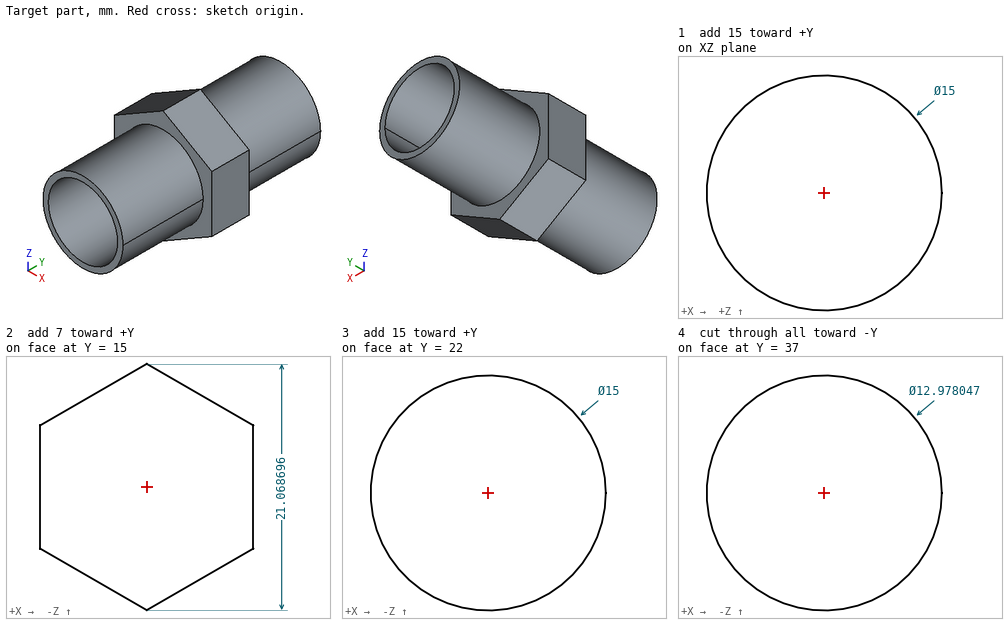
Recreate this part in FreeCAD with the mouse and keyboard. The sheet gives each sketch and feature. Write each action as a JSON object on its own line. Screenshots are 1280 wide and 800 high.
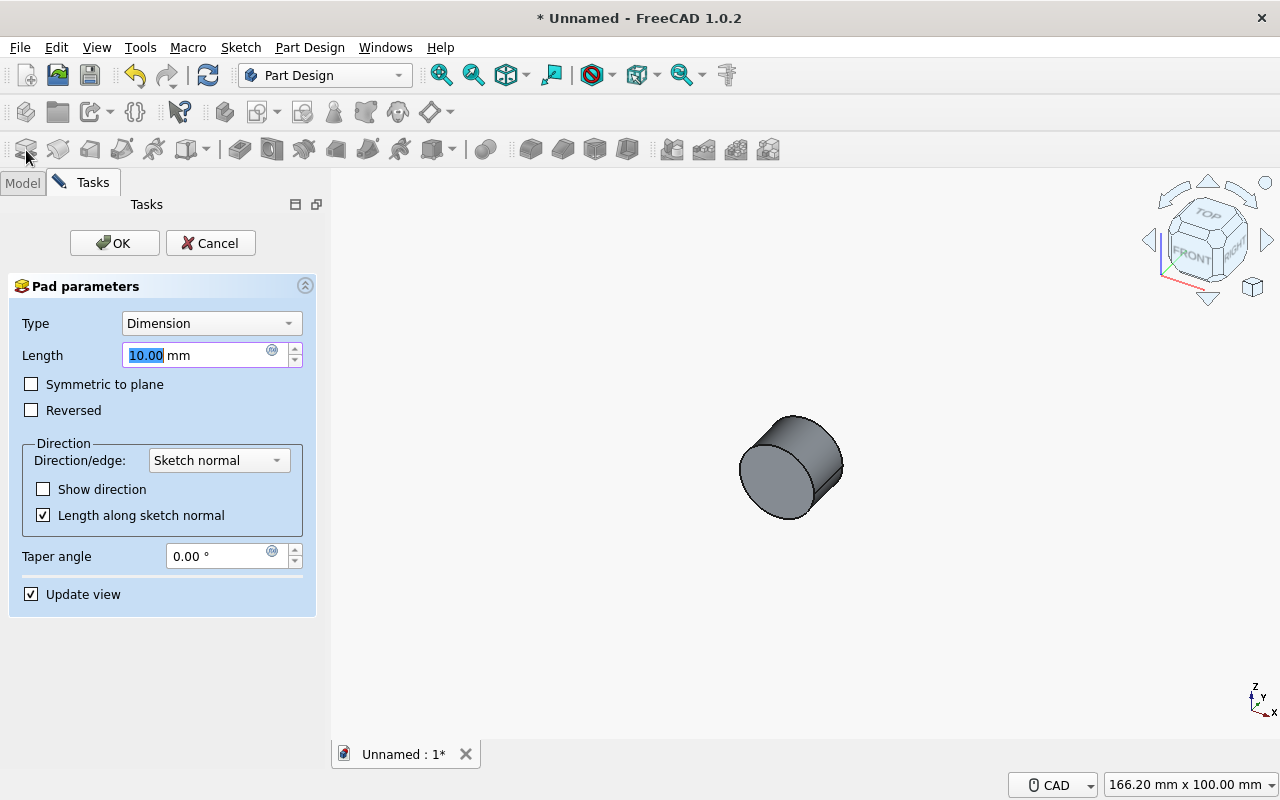
{"action": "type", "text": "15"}
{"action": "key", "text": "Tab"}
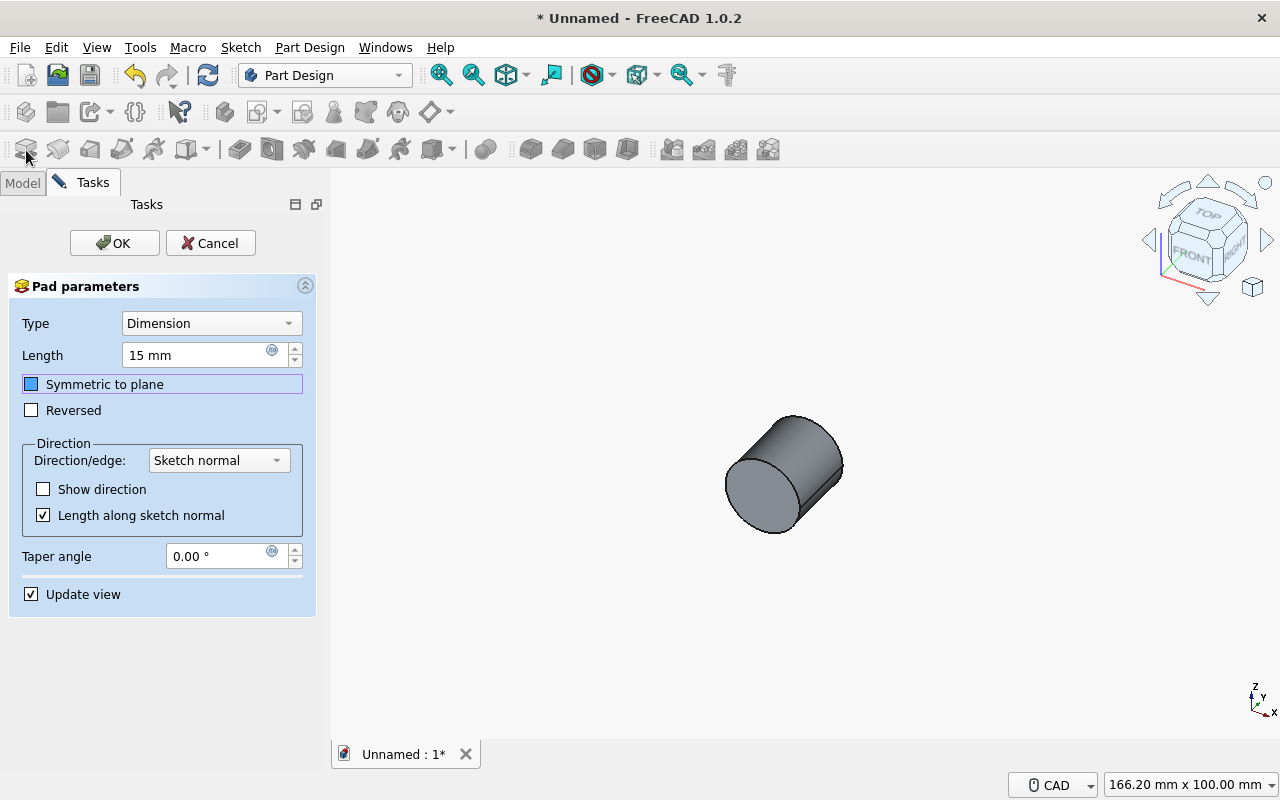
{"action": "left_click", "coordinate": [30, 410]}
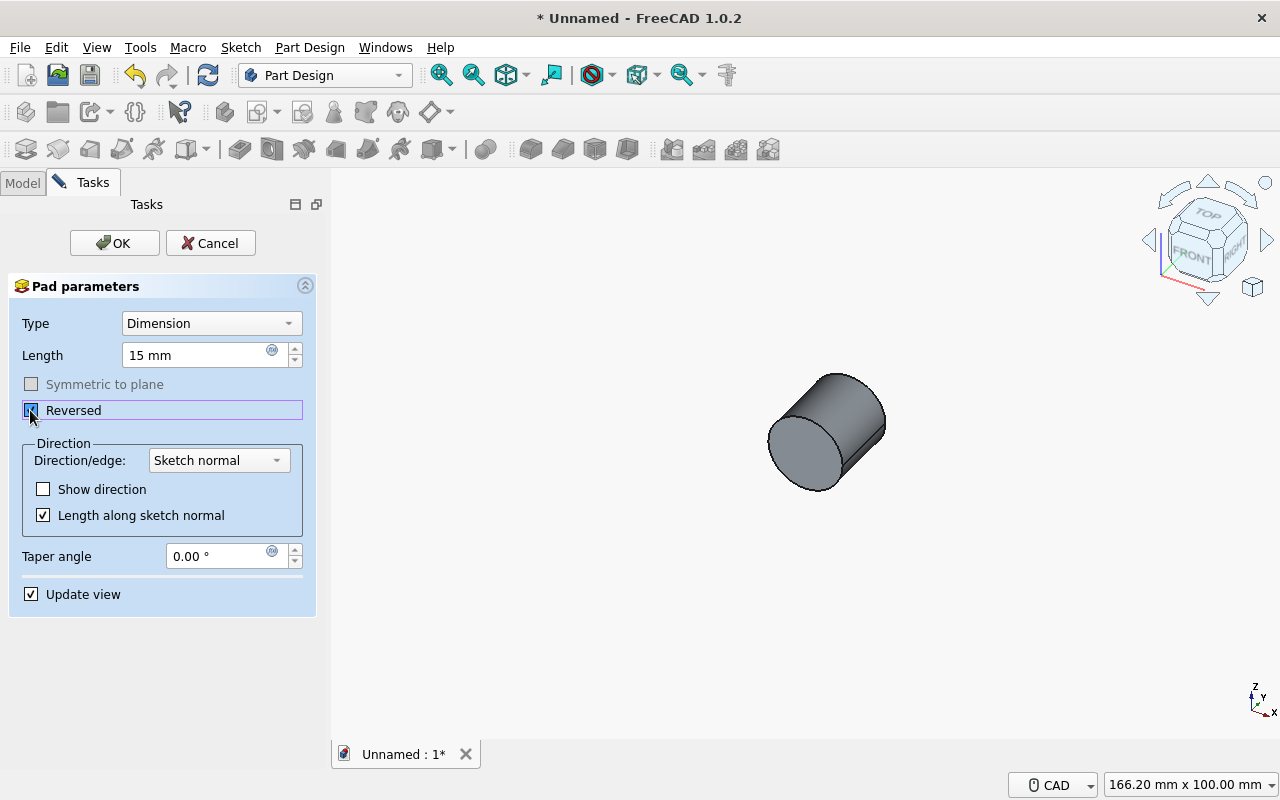
{"action": "left_click", "coordinate": [115, 243]}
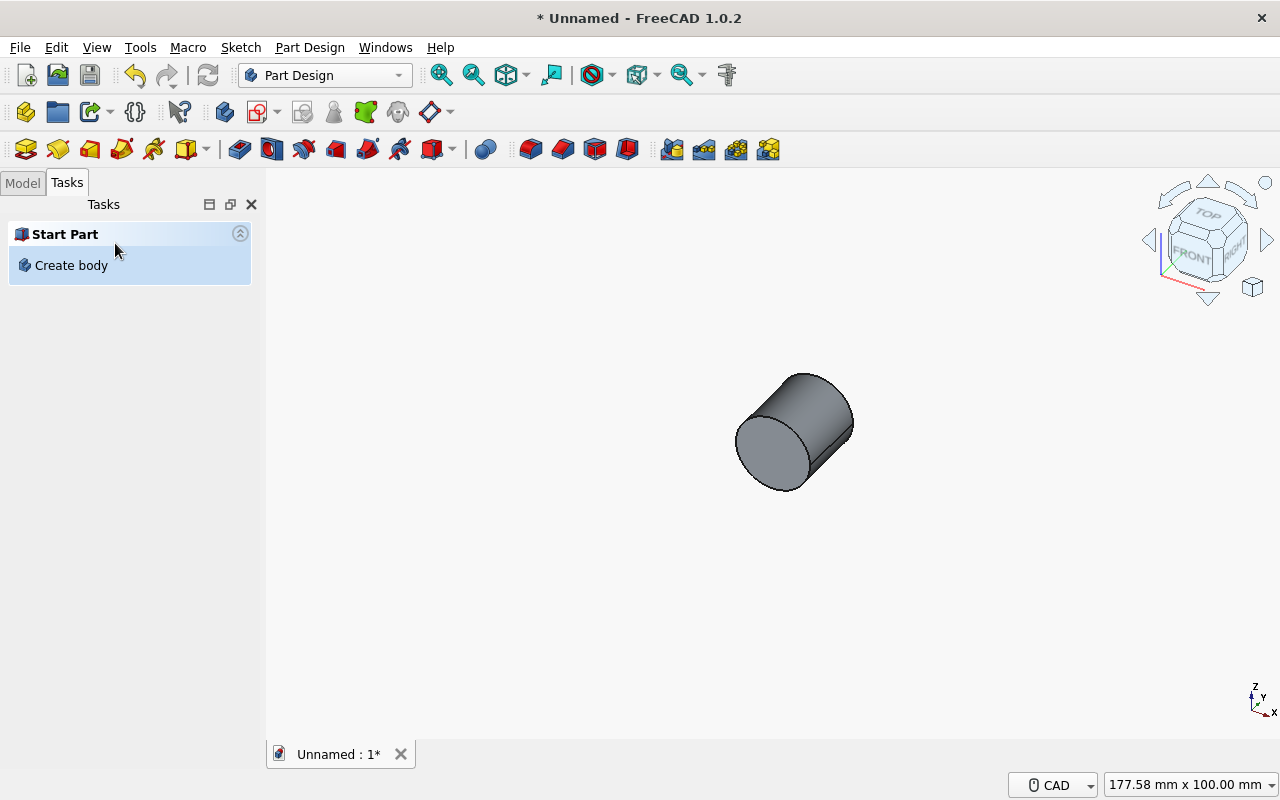
{"action": "left_click", "coordinate": [442, 76]}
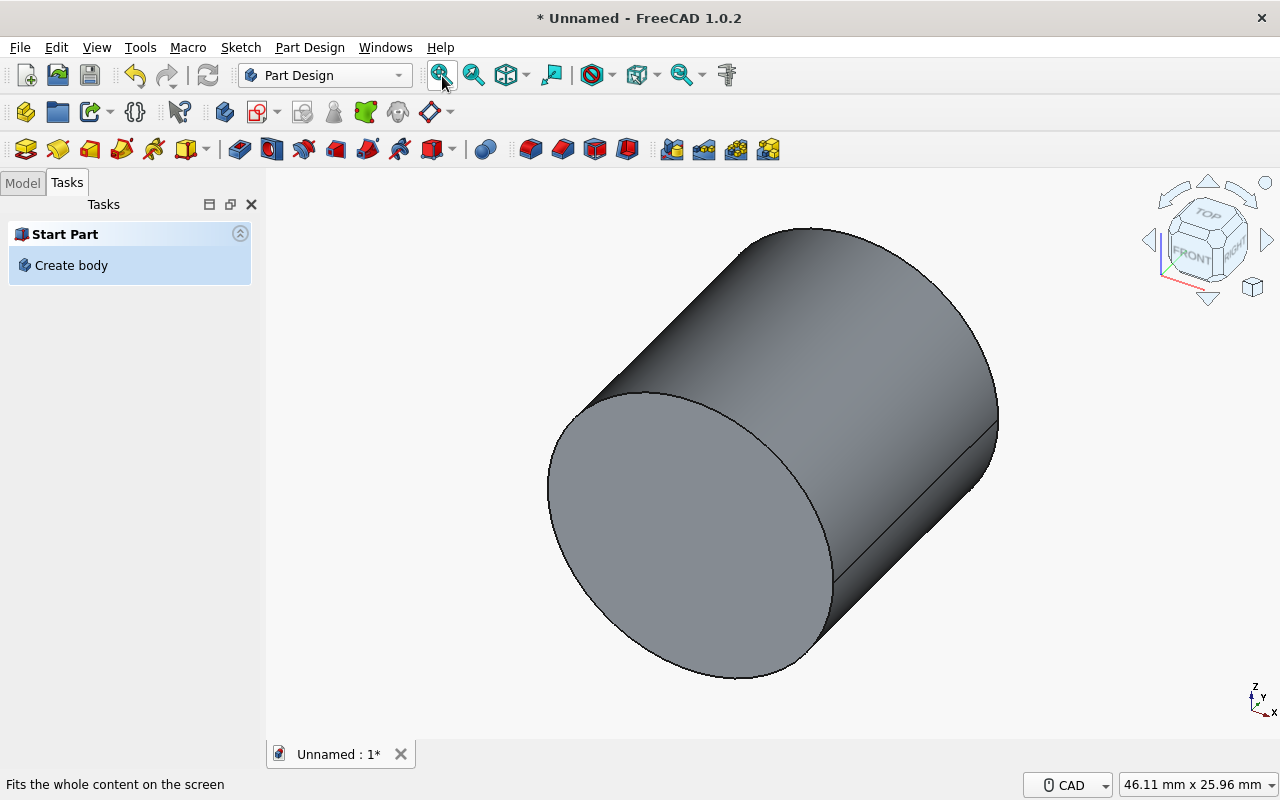
{"action": "key", "text": "4"}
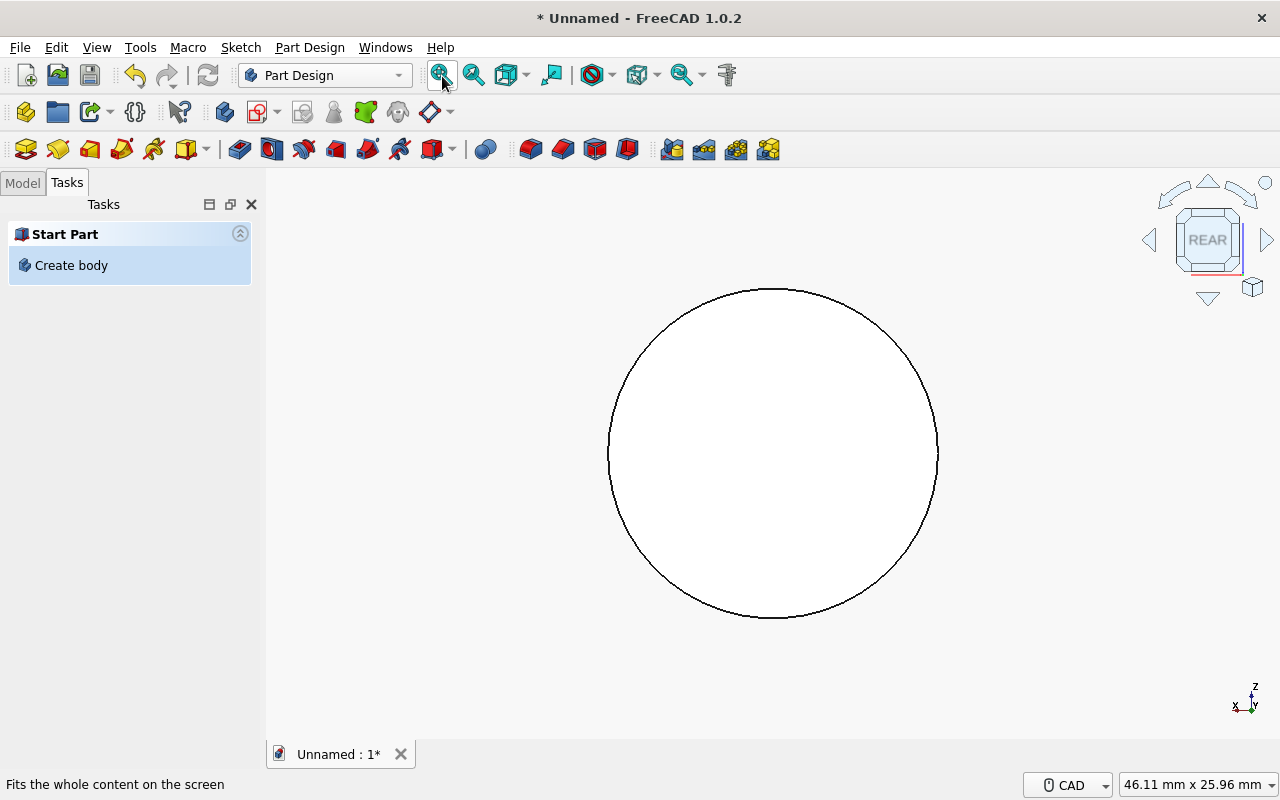
{"action": "left_click", "coordinate": [773, 453]}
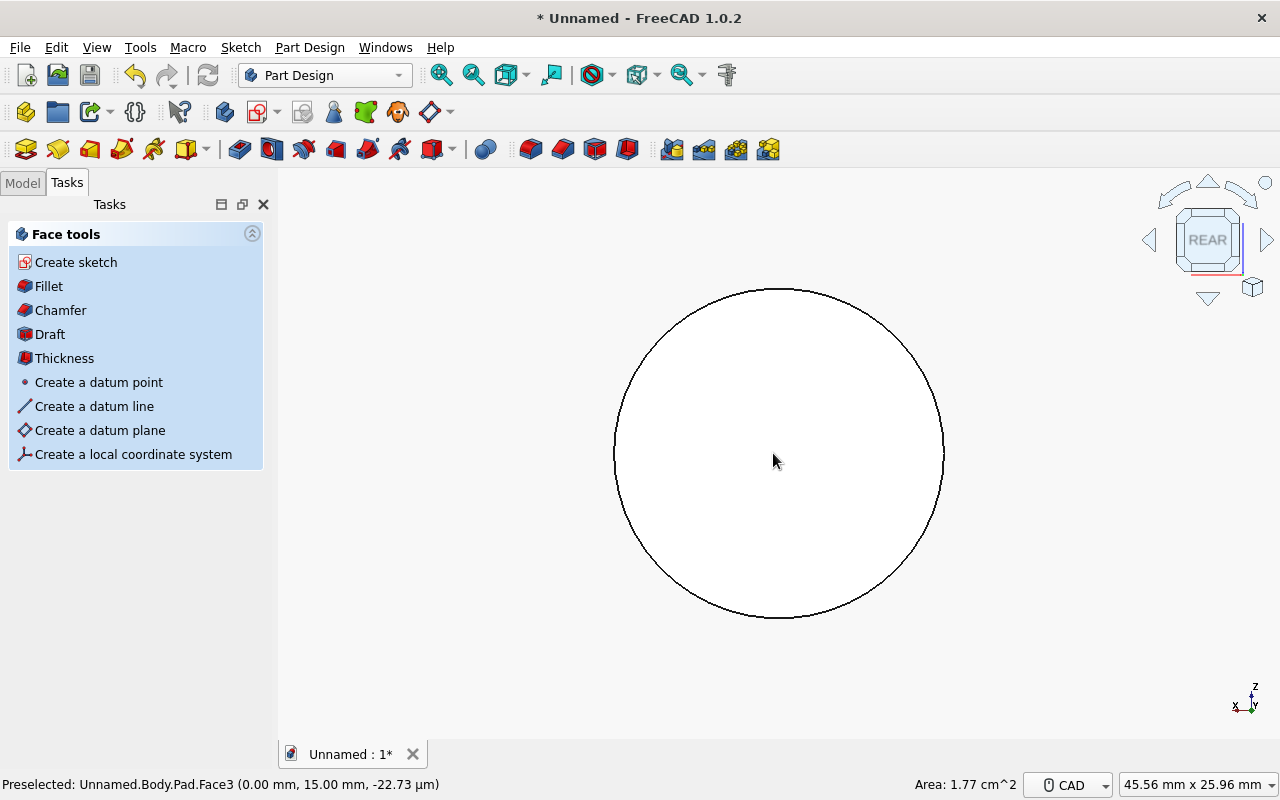
{"action": "left_click", "coordinate": [258, 112]}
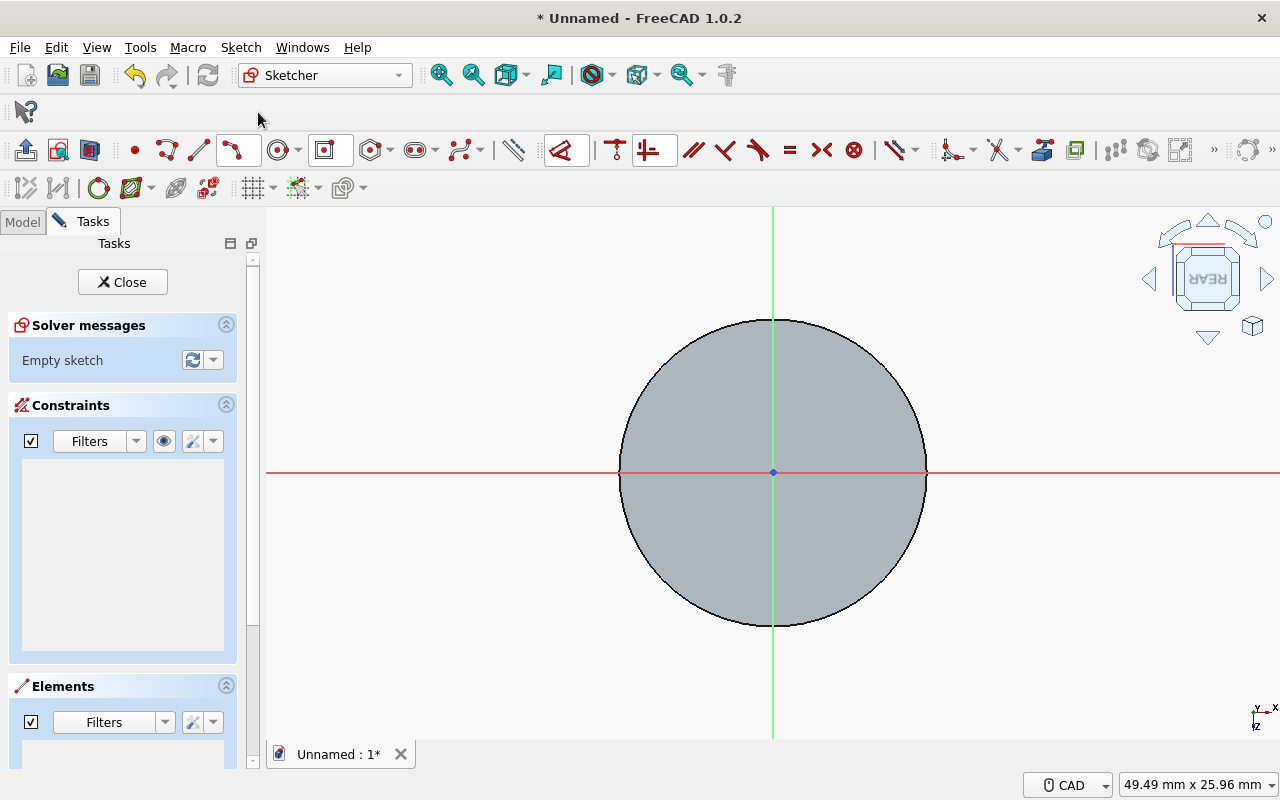
{"action": "scroll", "coordinate": [395, 473], "scroll_direction": "down", "scroll_amount": 1}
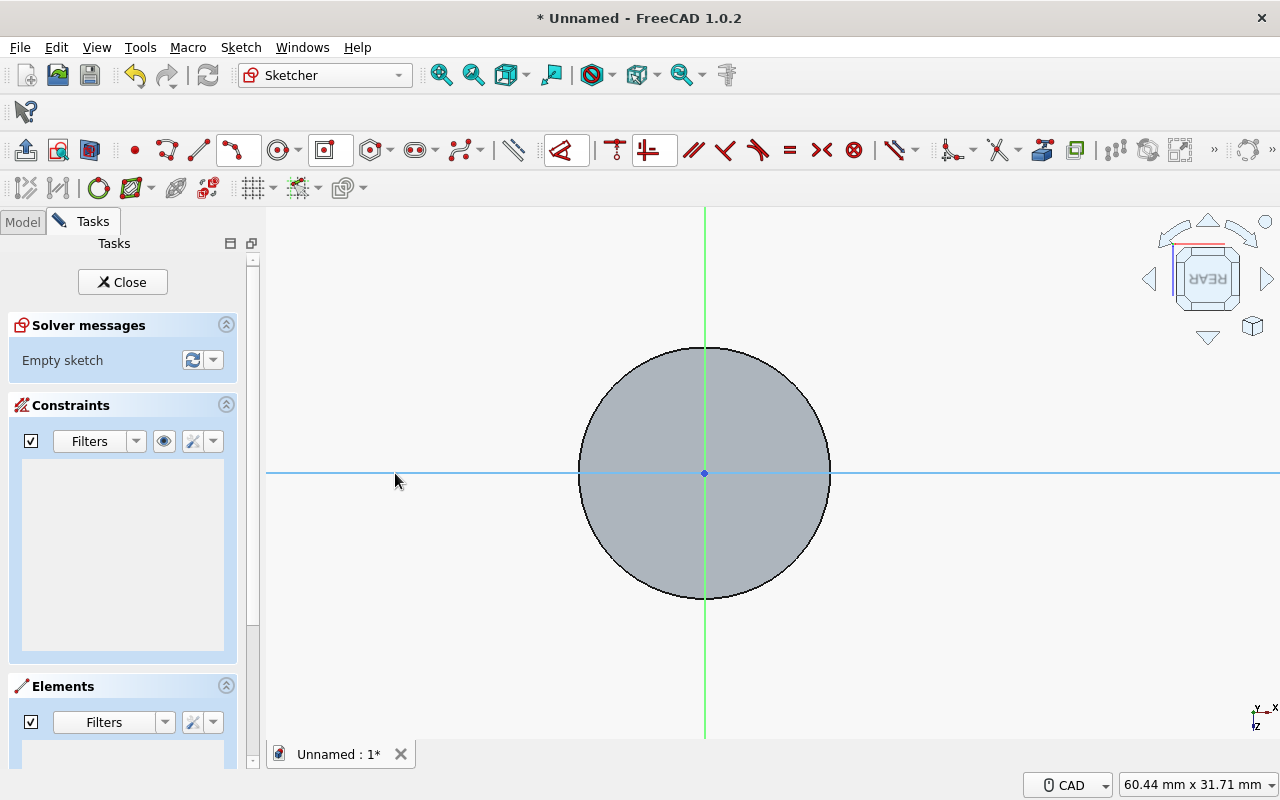
{"action": "left_click", "coordinate": [370, 150]}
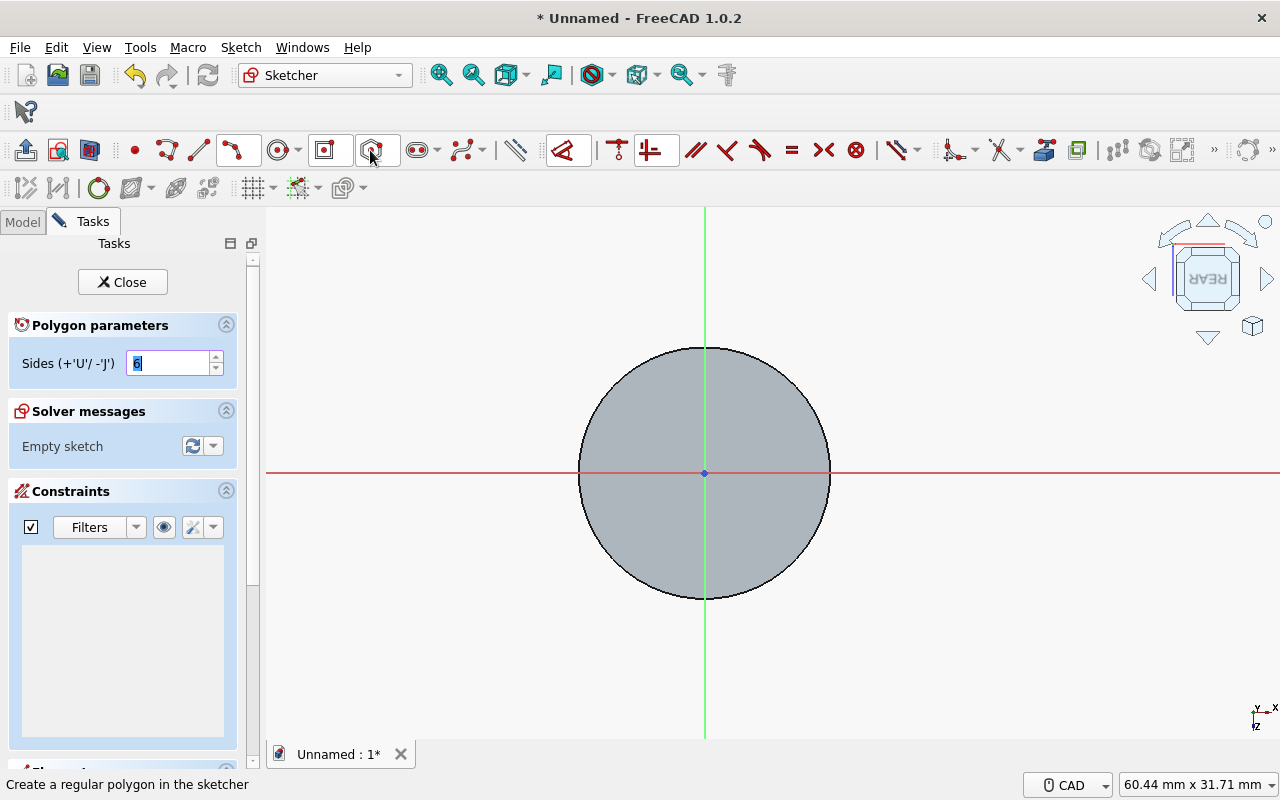
{"action": "left_click", "coordinate": [705, 473]}